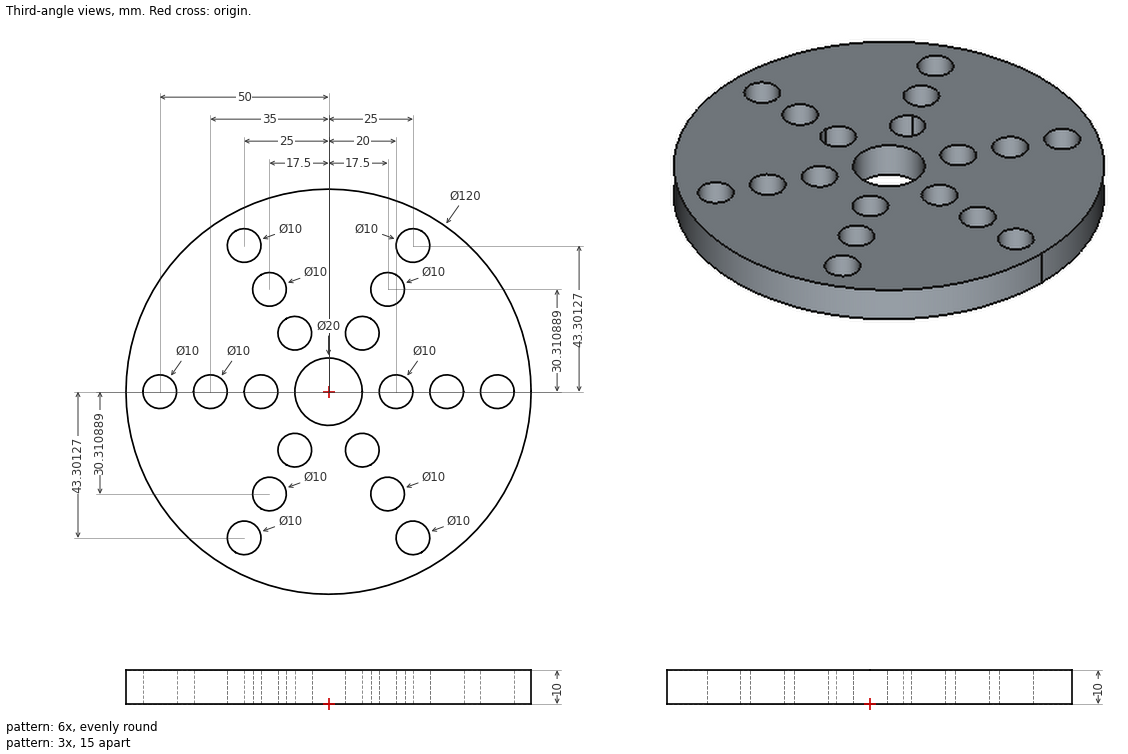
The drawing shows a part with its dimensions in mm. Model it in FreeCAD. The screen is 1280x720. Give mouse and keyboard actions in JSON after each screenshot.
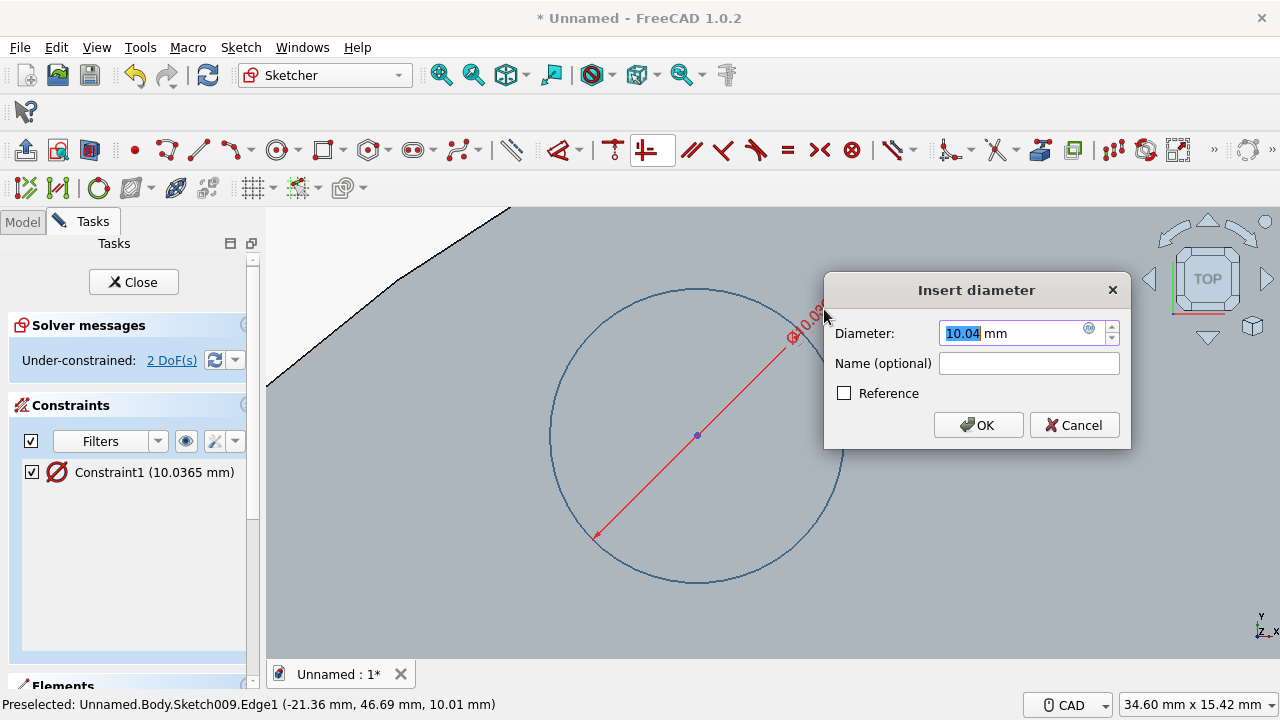
{"action": "type", "text": "10"}
{"action": "key", "text": "Return"}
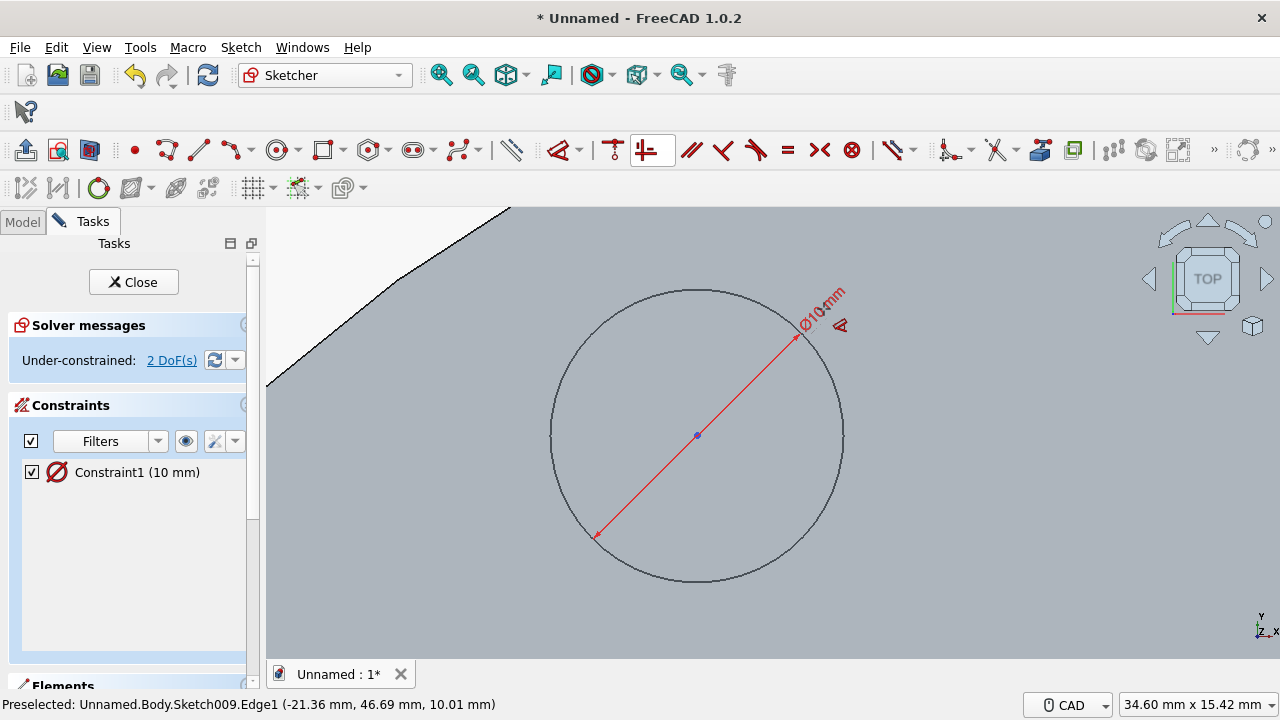
{"action": "left_click", "coordinate": [697, 436]}
{"action": "left_click", "coordinate": [906, 402]}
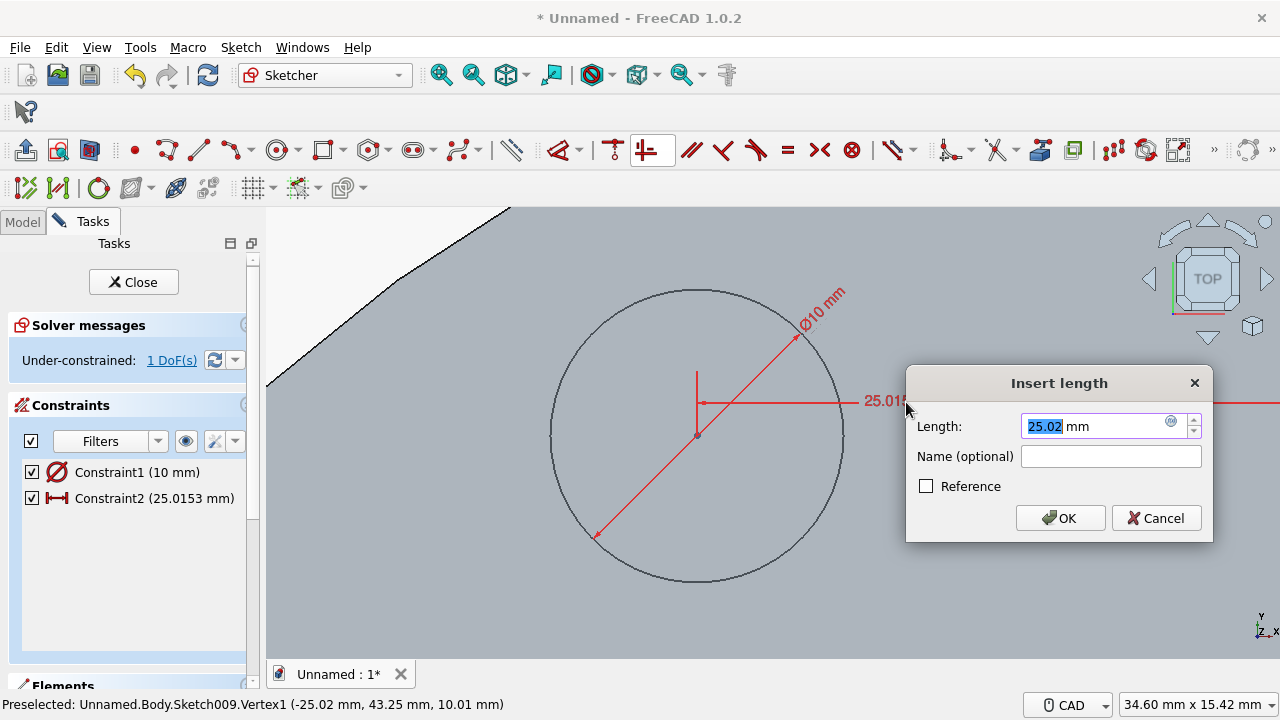
{"action": "type", "text": "25"}
{"action": "key", "text": "Return"}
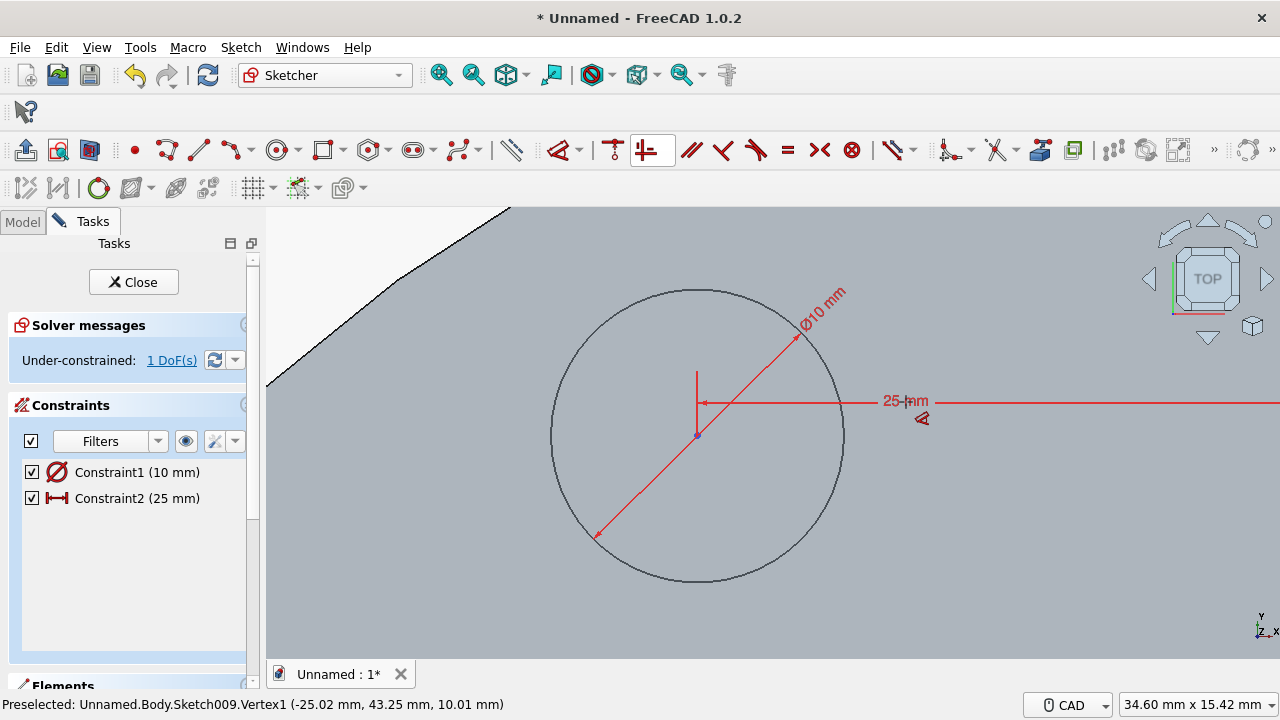
{"action": "left_click", "coordinate": [697, 436]}
{"action": "left_click", "coordinate": [663, 534]}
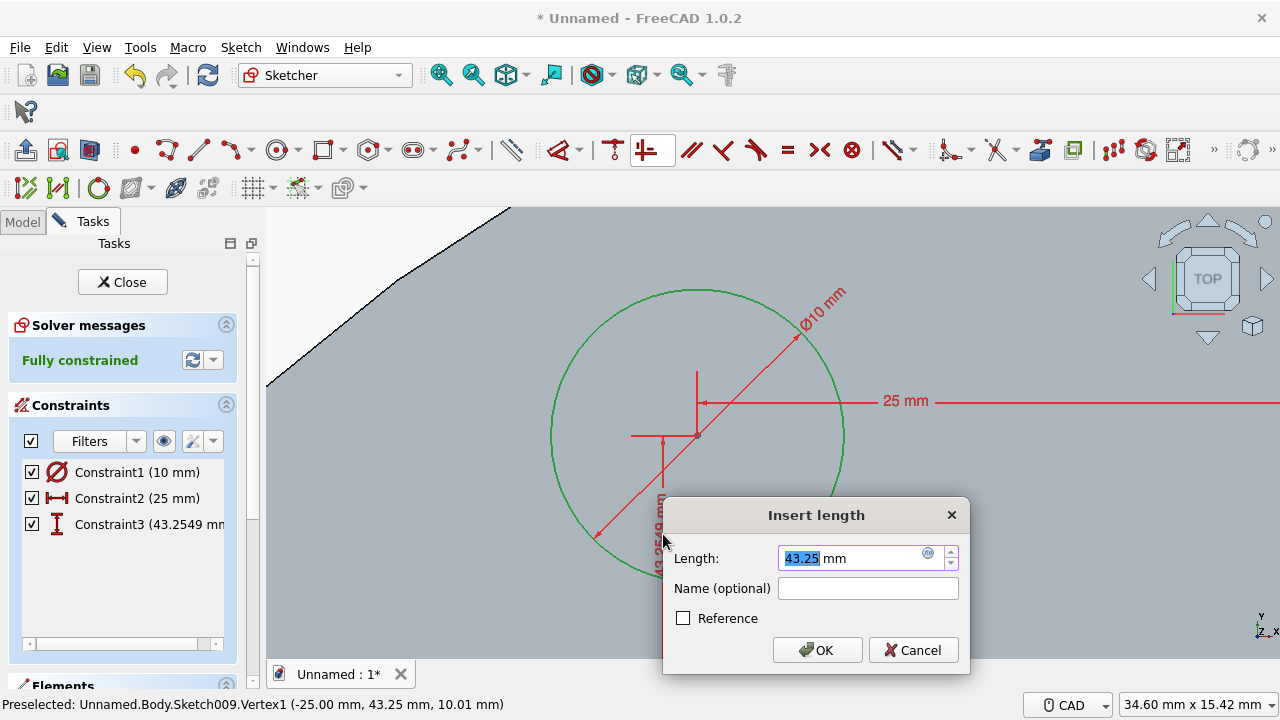
{"action": "type", "text": "43.30127"}
{"action": "key", "text": "Return"}
{"action": "key", "text": "Escape"}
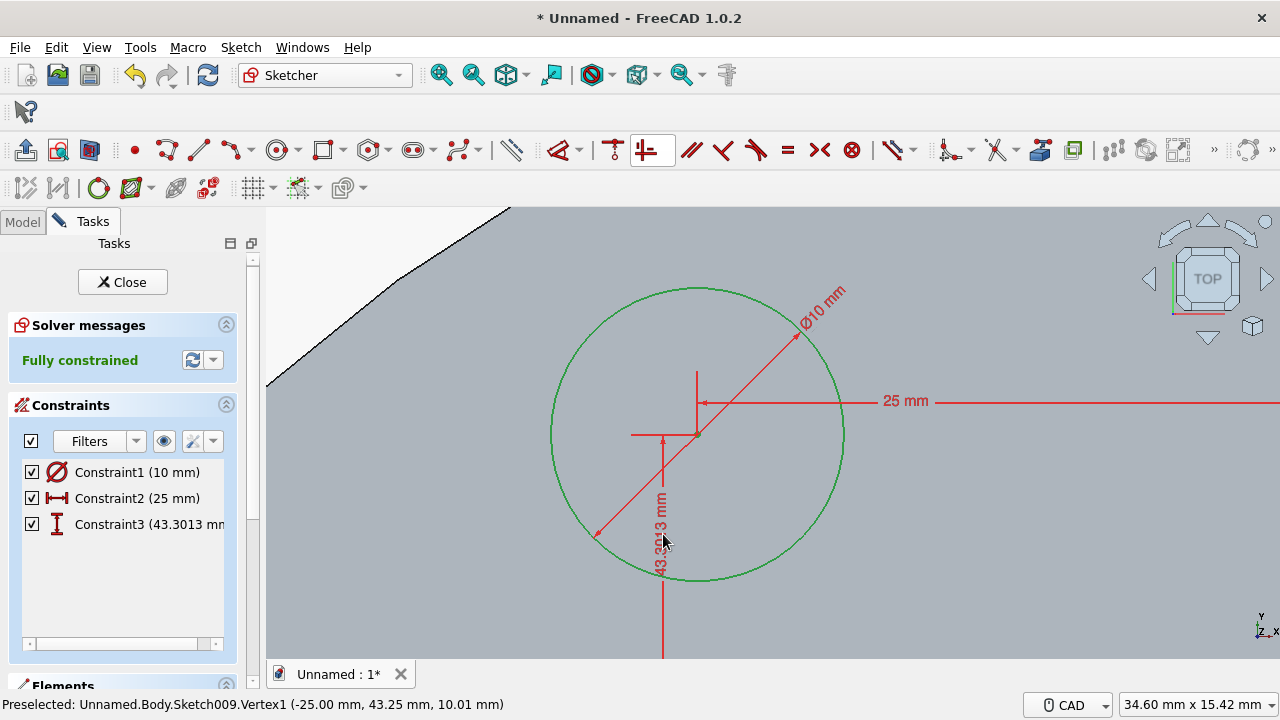
{"action": "left_click", "coordinate": [123, 282]}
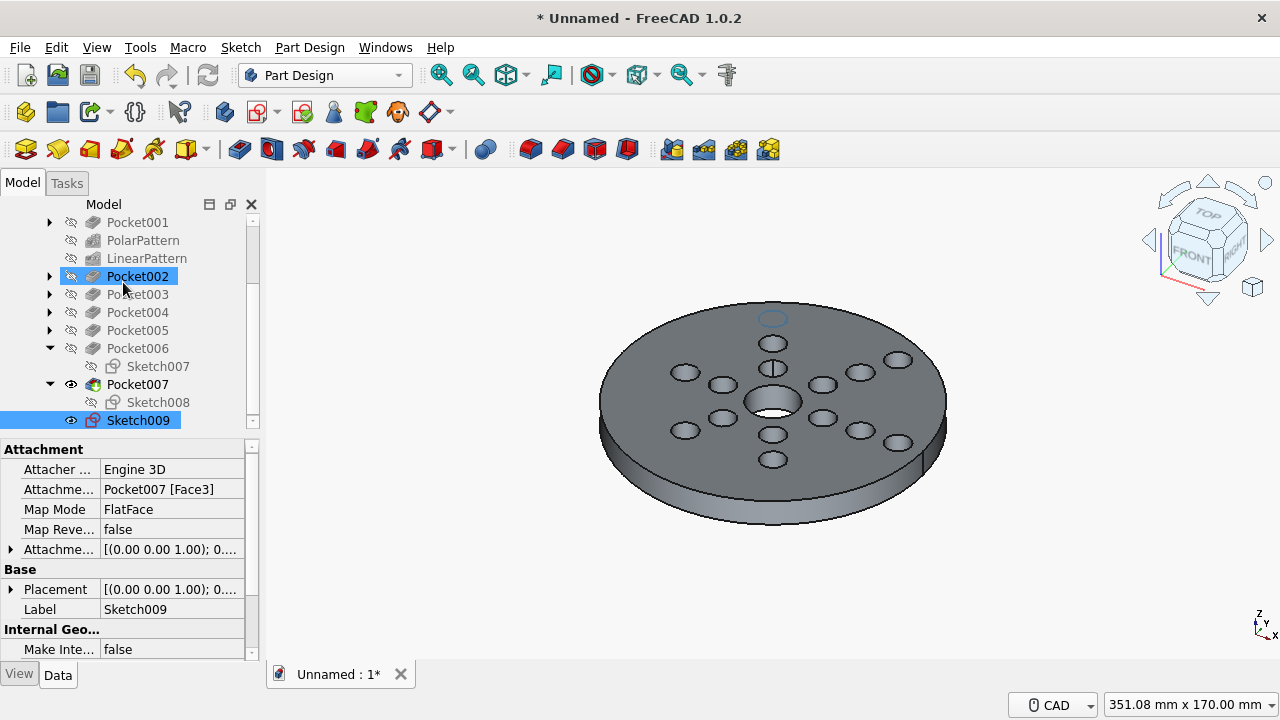
{"action": "left_click", "coordinate": [240, 150]}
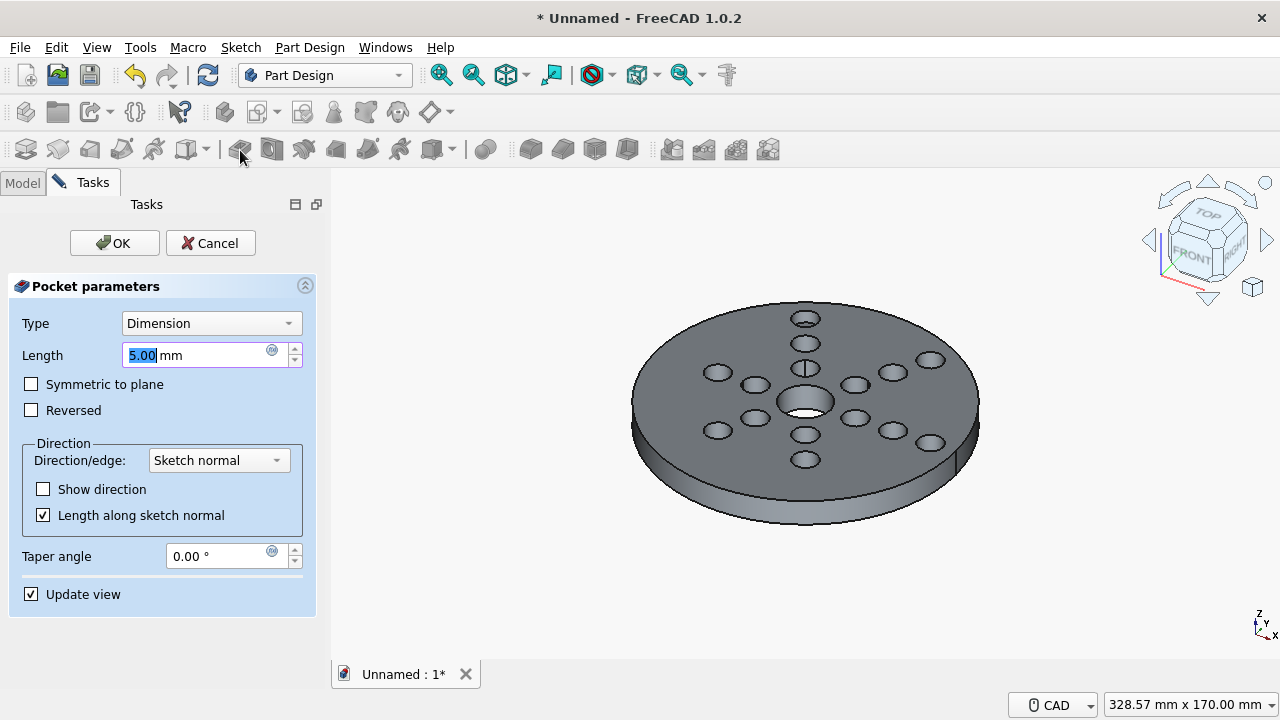
{"action": "type", "text": "10"}
{"action": "key", "text": "Tab"}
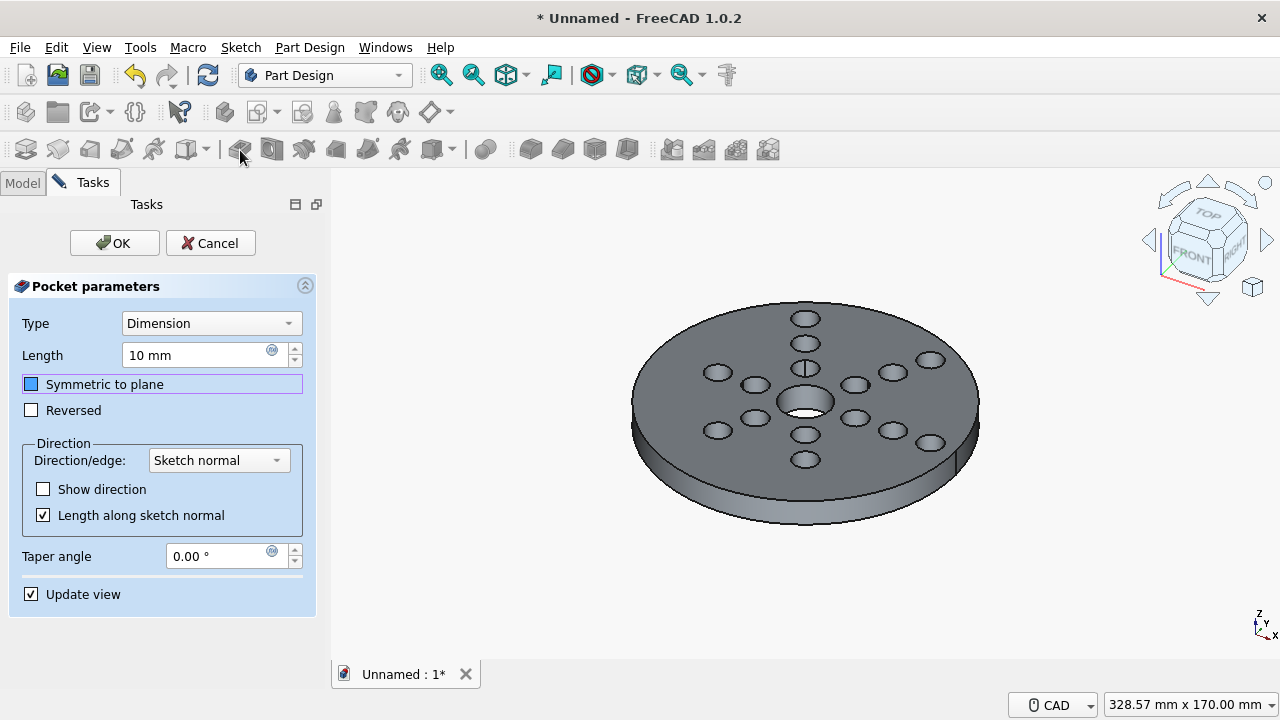
{"action": "left_click", "coordinate": [115, 243]}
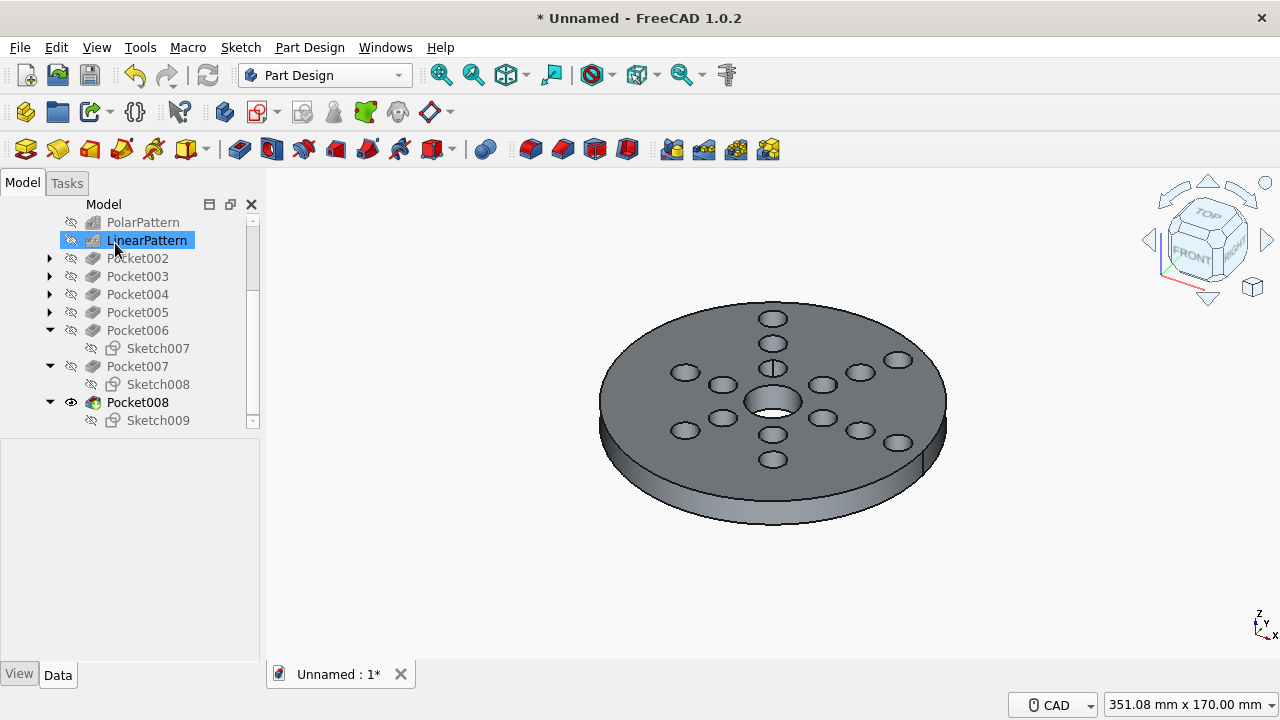
{"action": "left_click", "coordinate": [823, 351]}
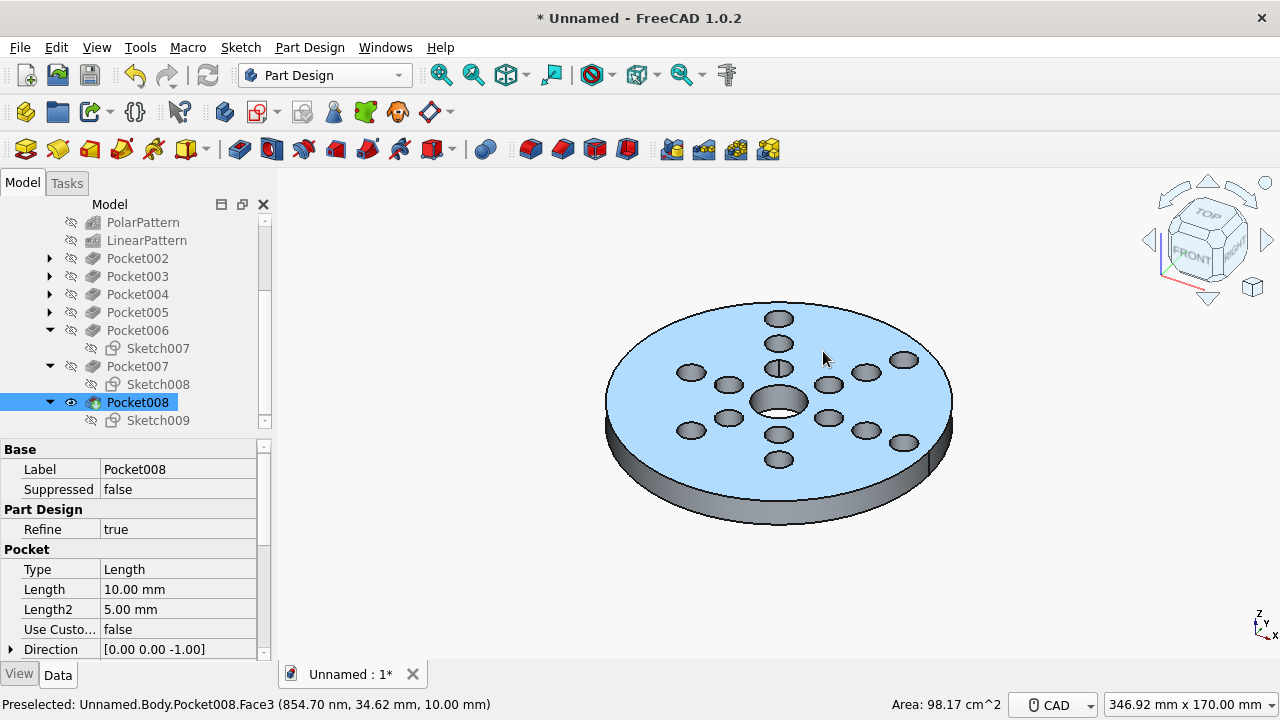
{"action": "left_click", "coordinate": [258, 112]}